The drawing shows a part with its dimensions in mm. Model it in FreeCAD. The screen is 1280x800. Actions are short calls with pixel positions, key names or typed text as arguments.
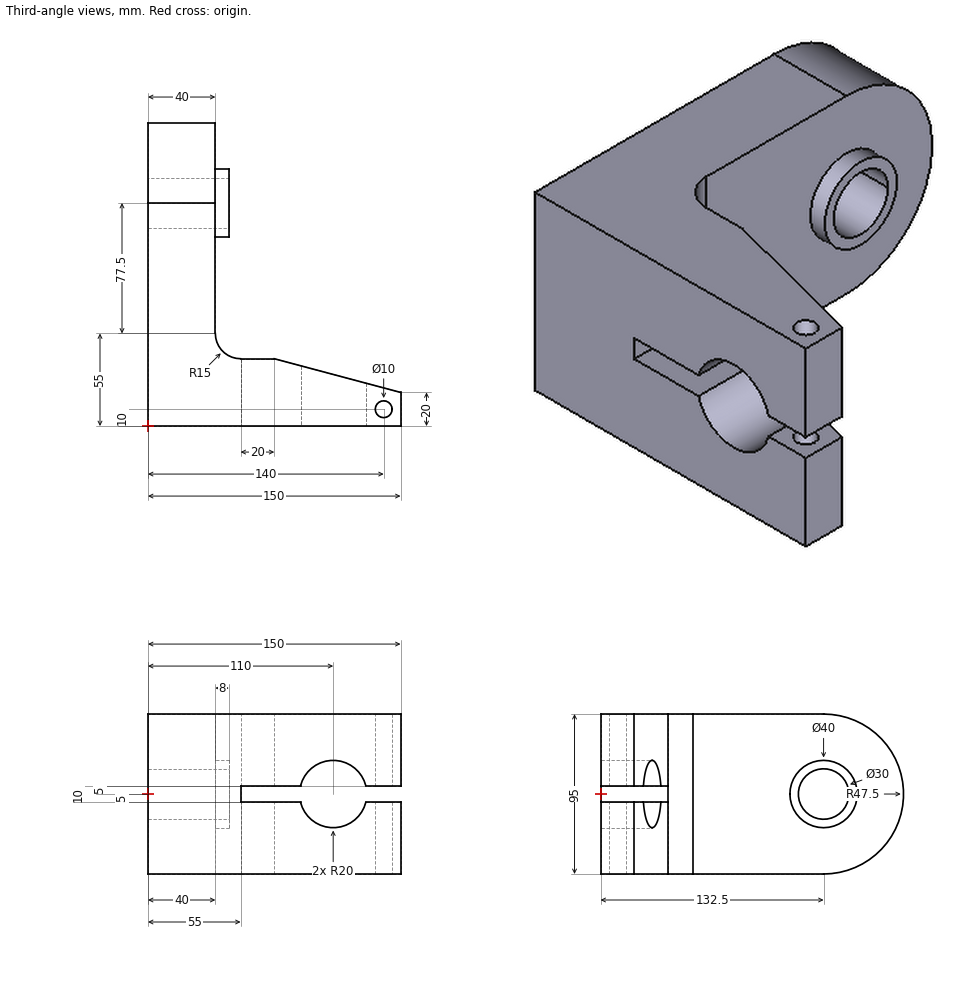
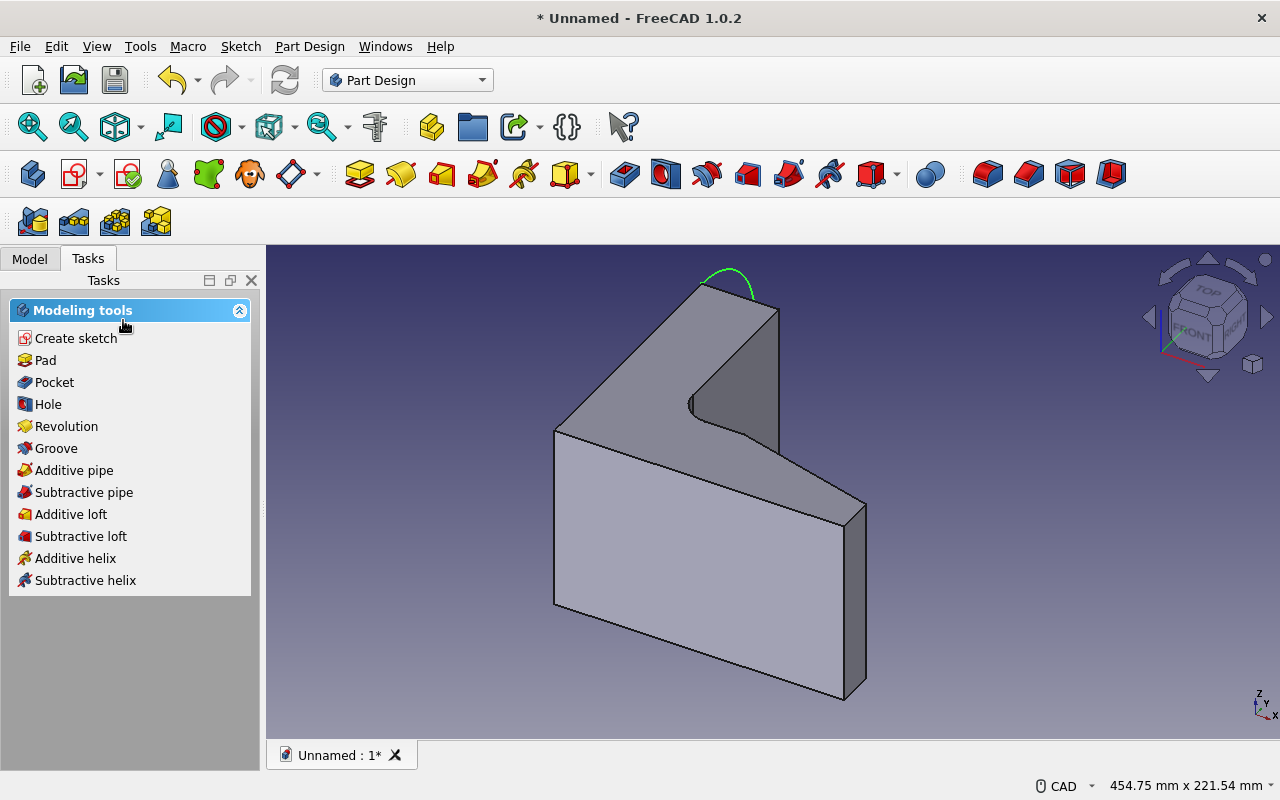
click(360, 174)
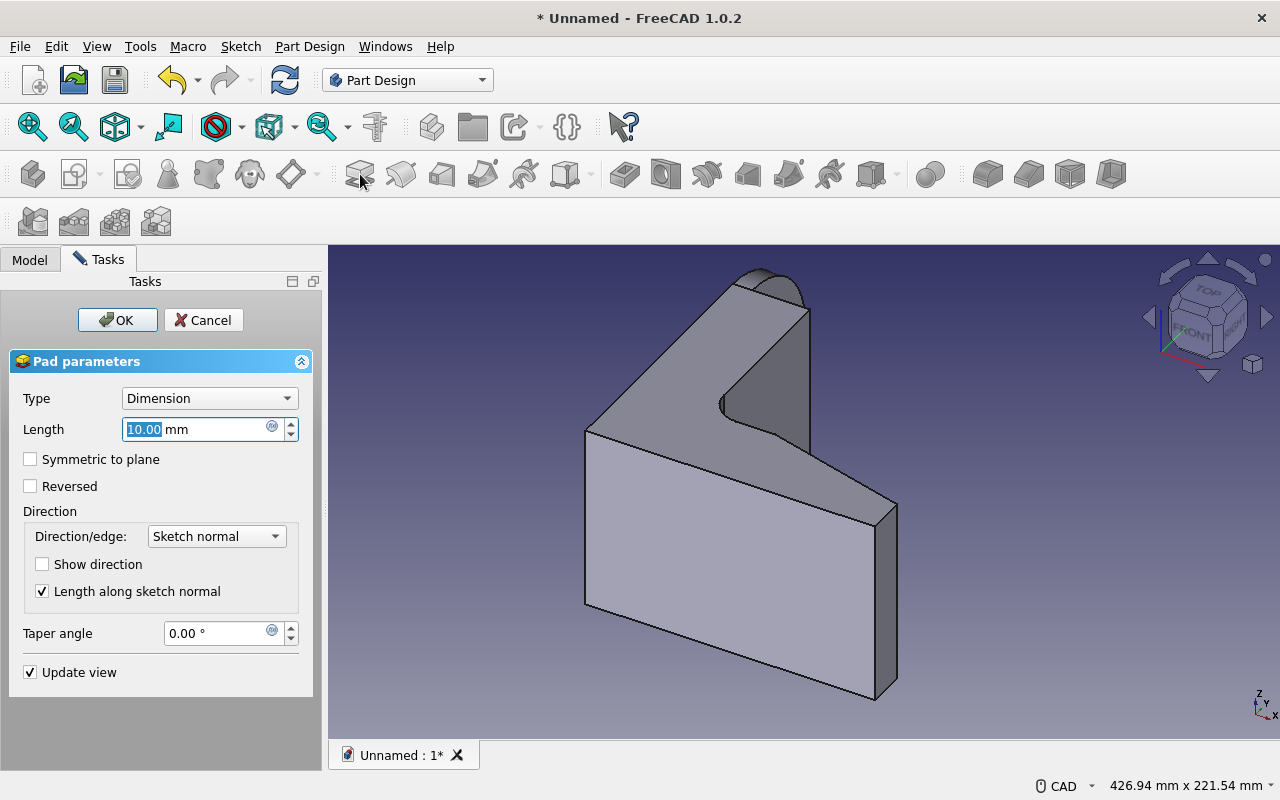
text(40)
key(Tab)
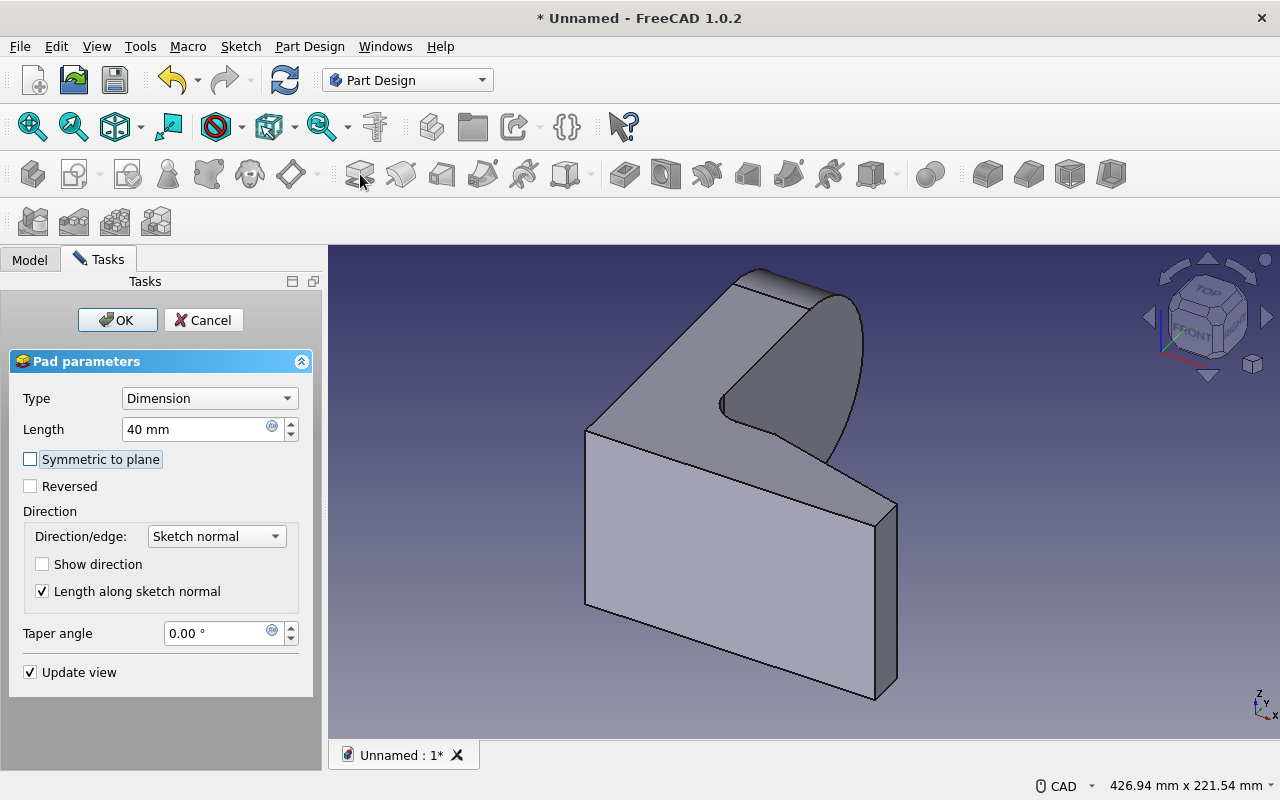
click(118, 320)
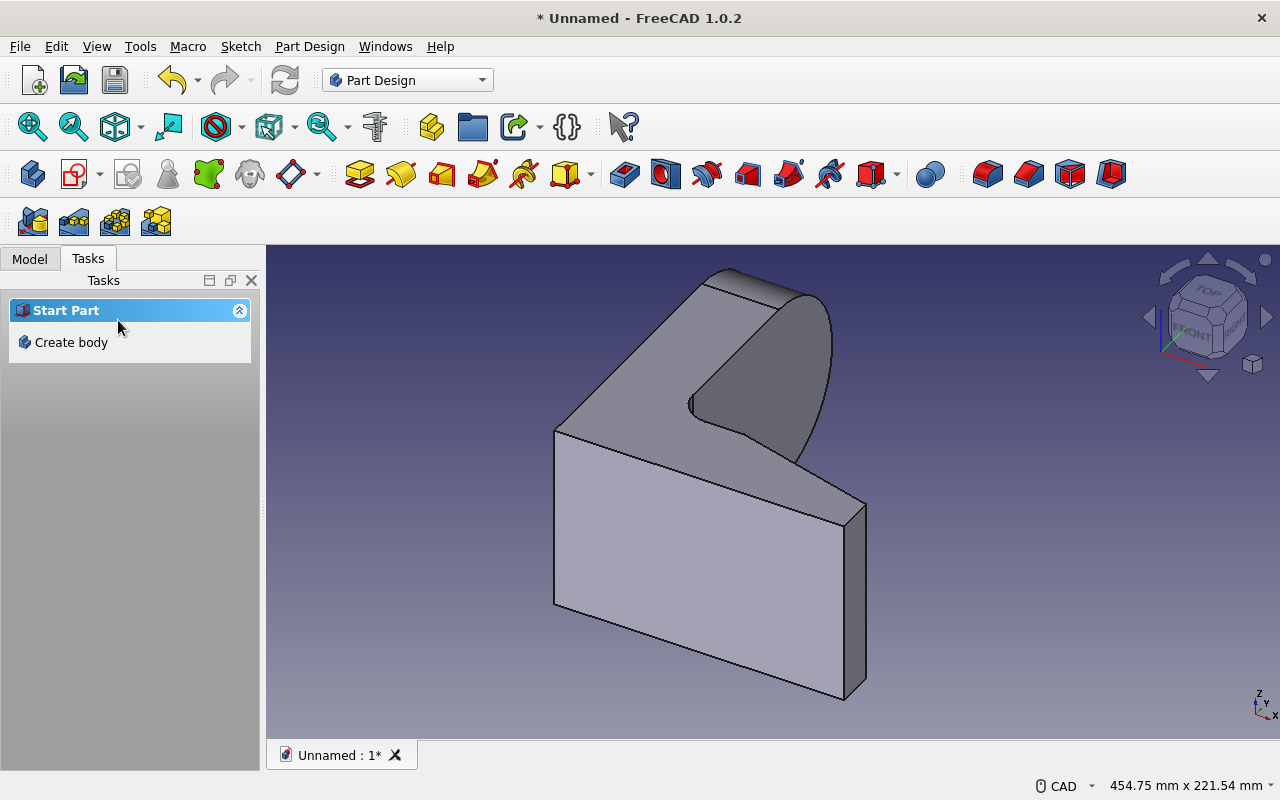
click(33, 128)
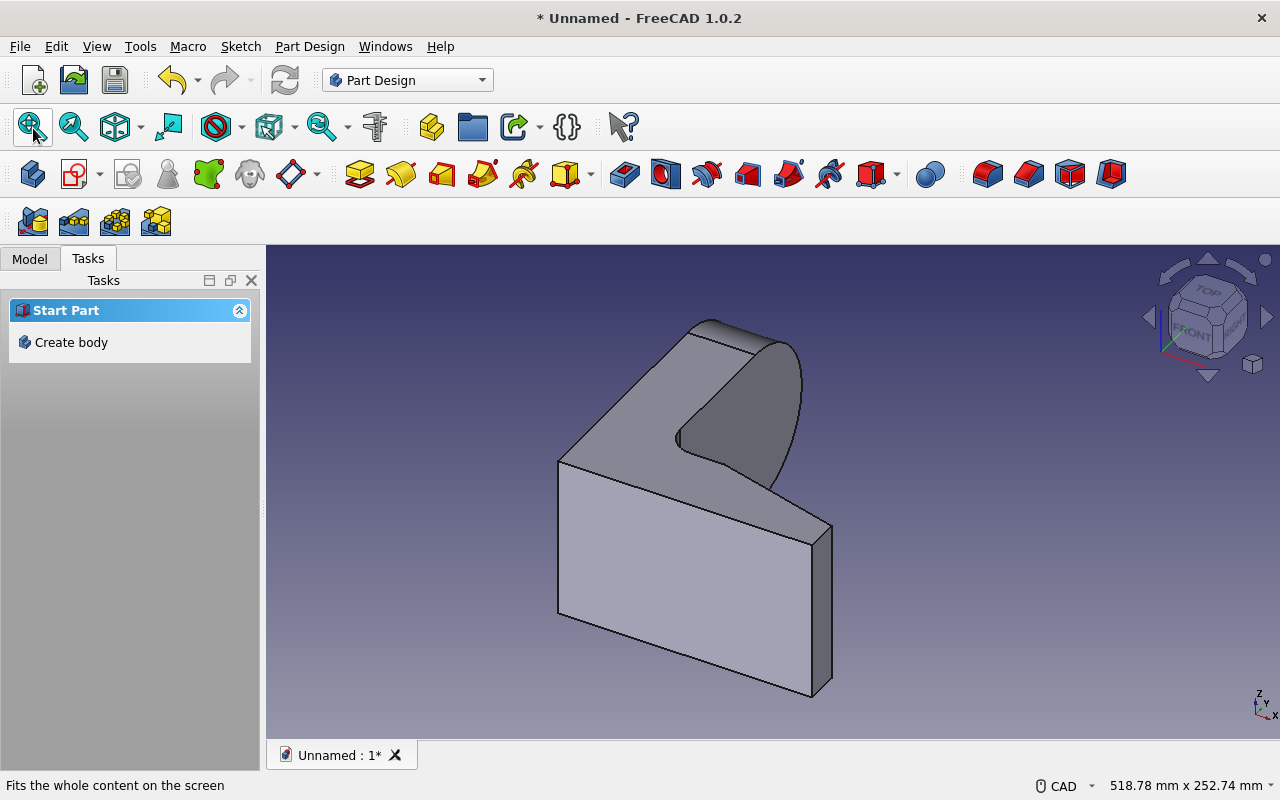
click(741, 445)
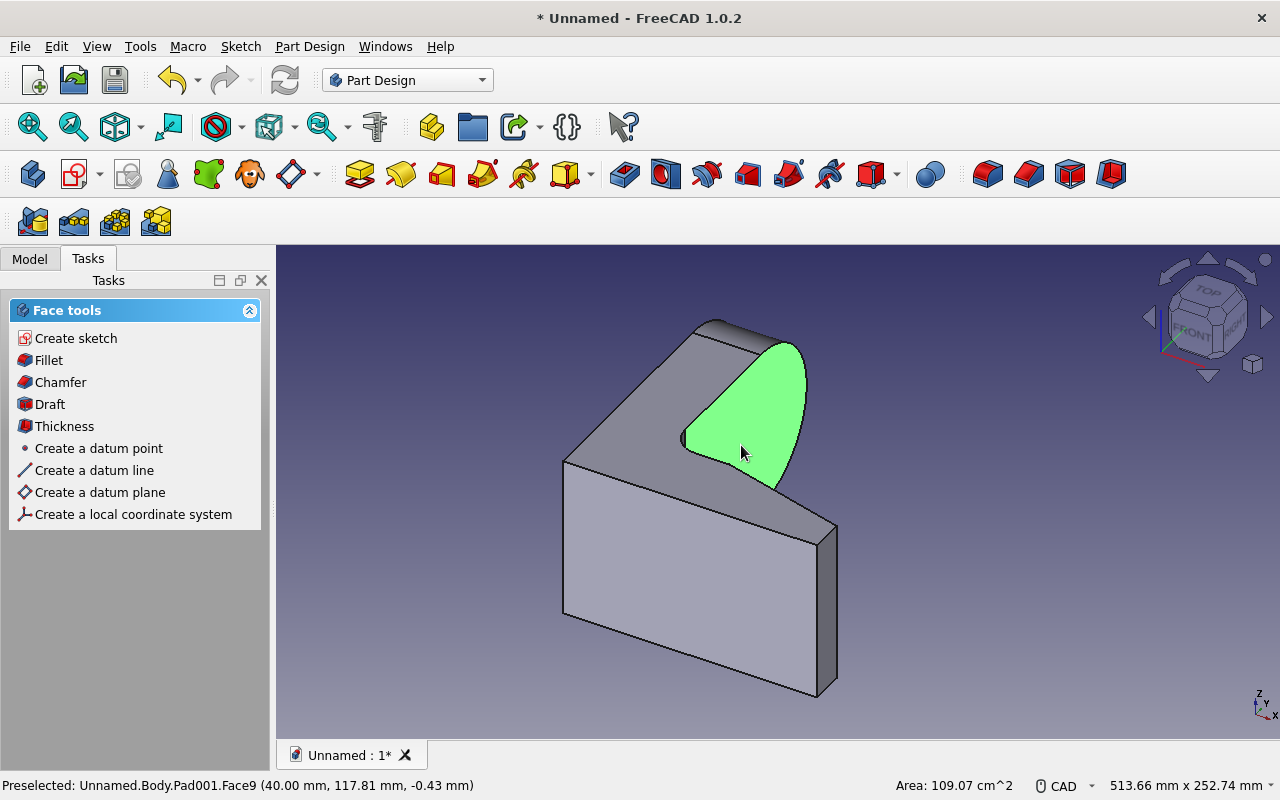
click(74, 174)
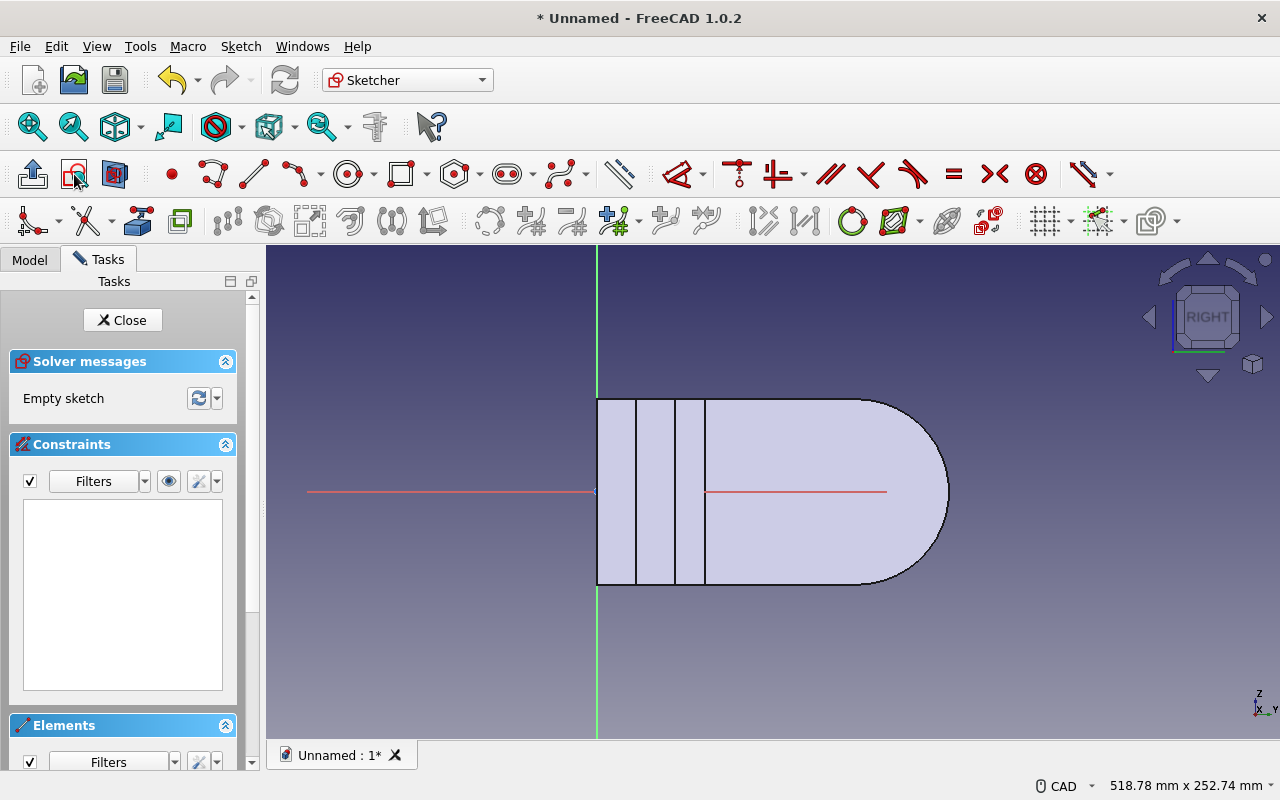
click(115, 174)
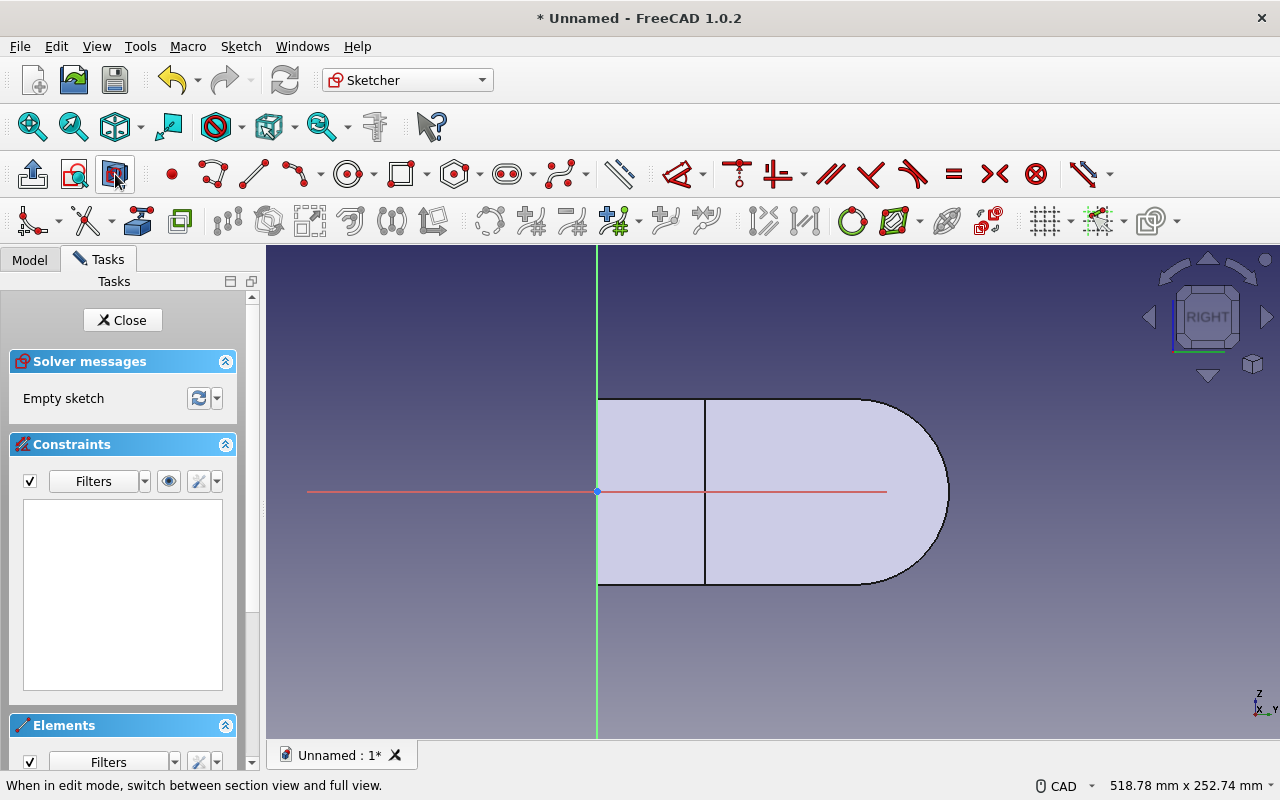
scroll(906, 492, up, 7)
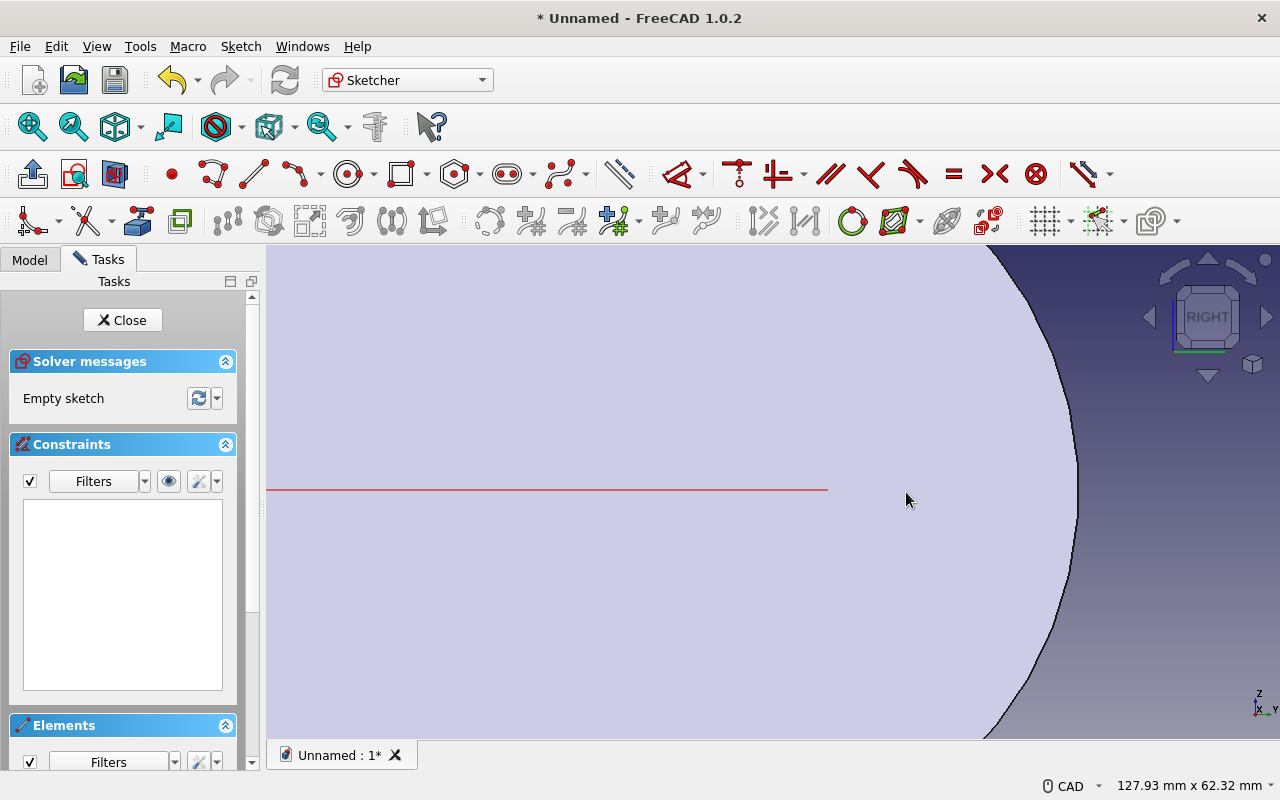
click(348, 174)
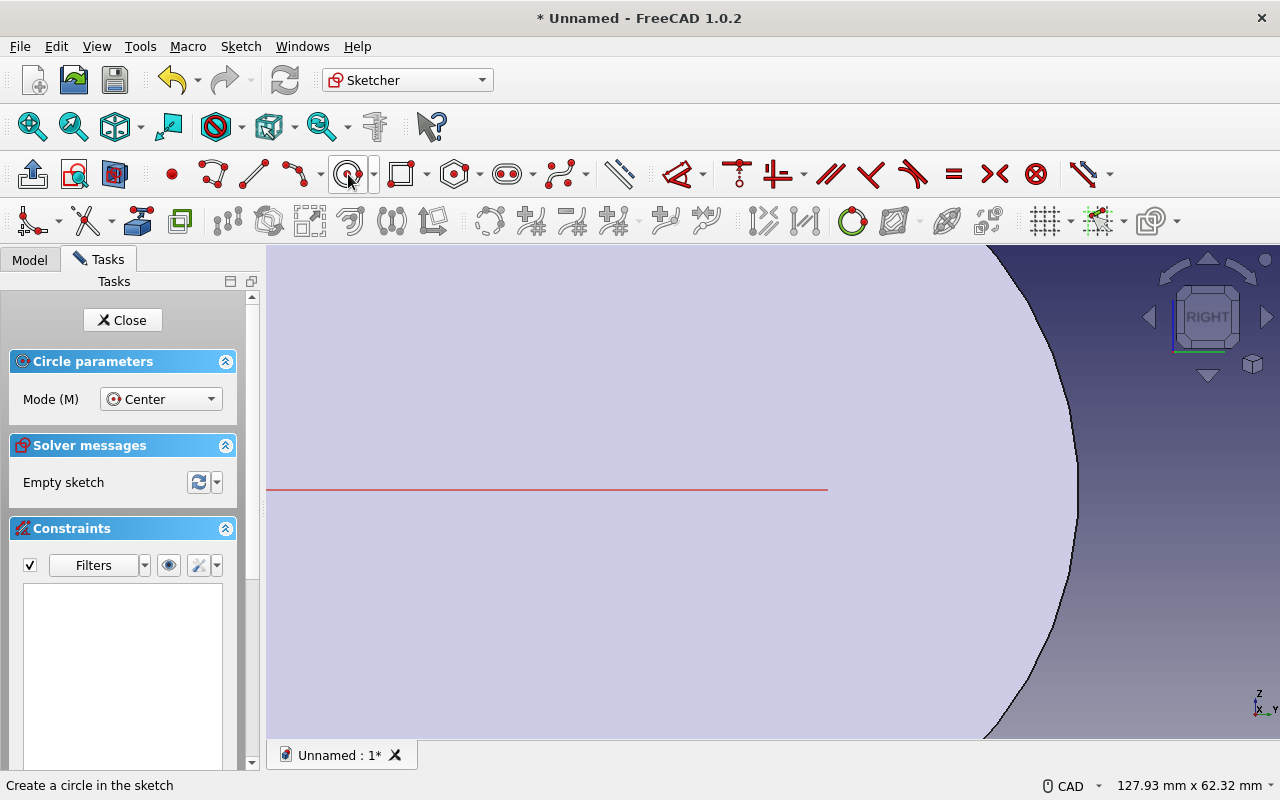
click(702, 490)
move(814, 378)